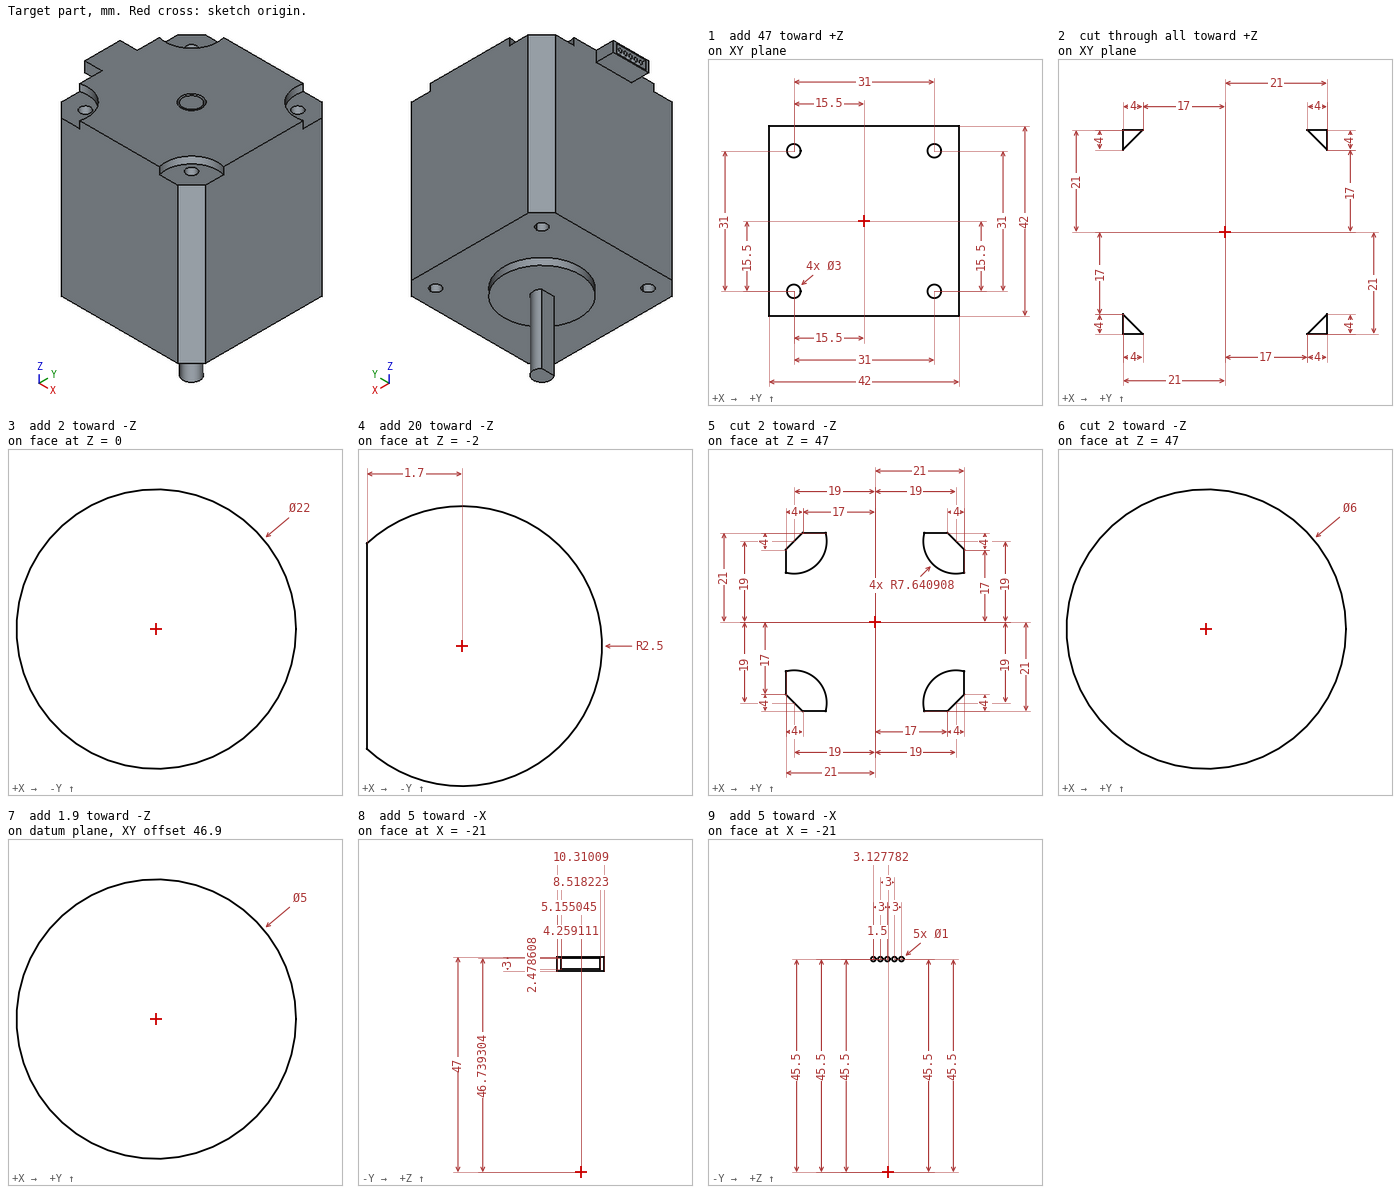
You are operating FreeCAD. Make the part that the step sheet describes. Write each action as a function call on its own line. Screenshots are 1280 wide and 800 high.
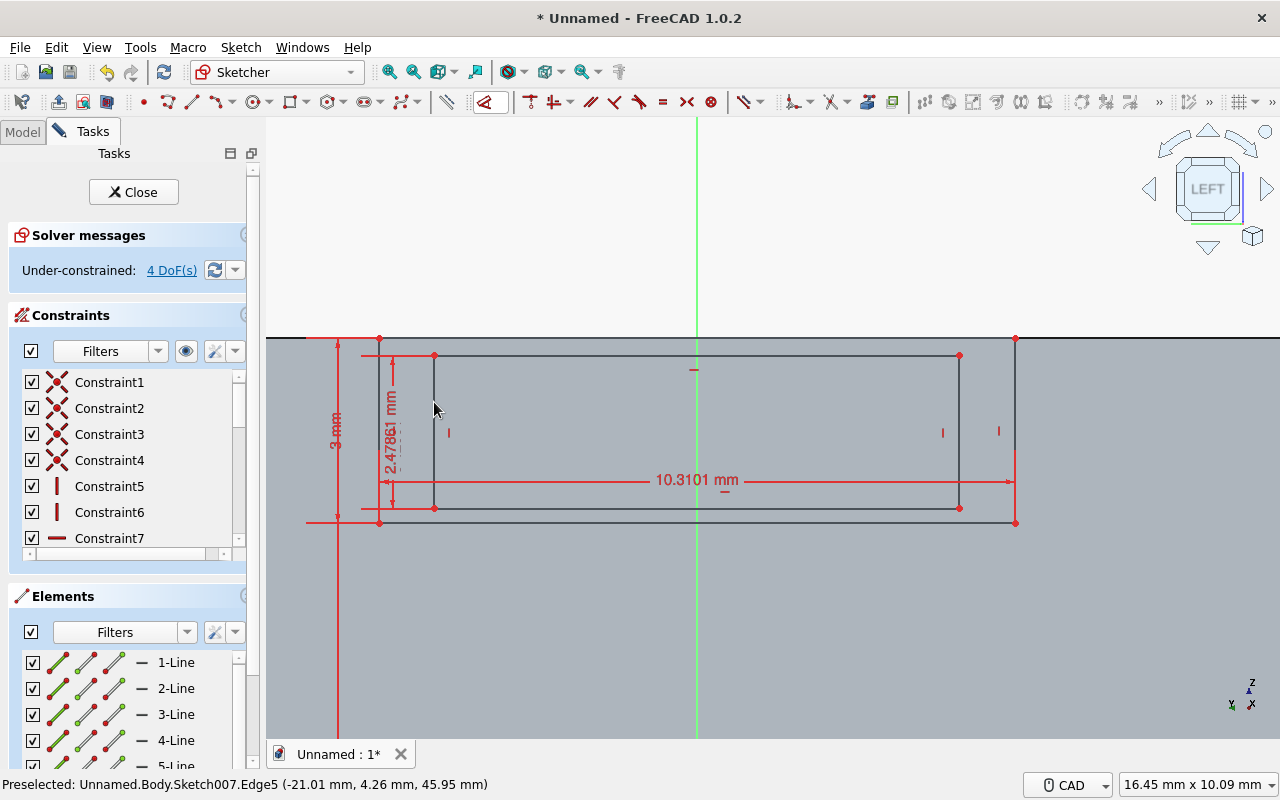
click(591, 509)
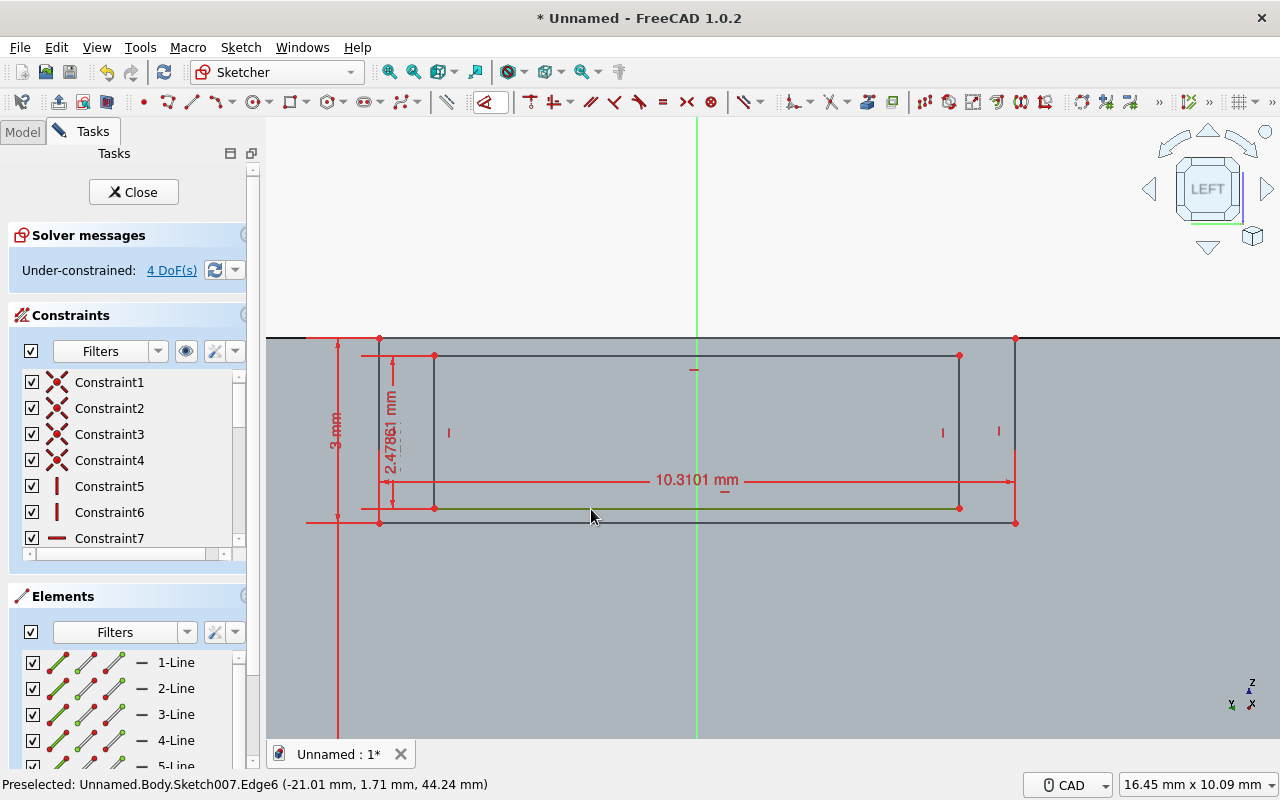
key(l)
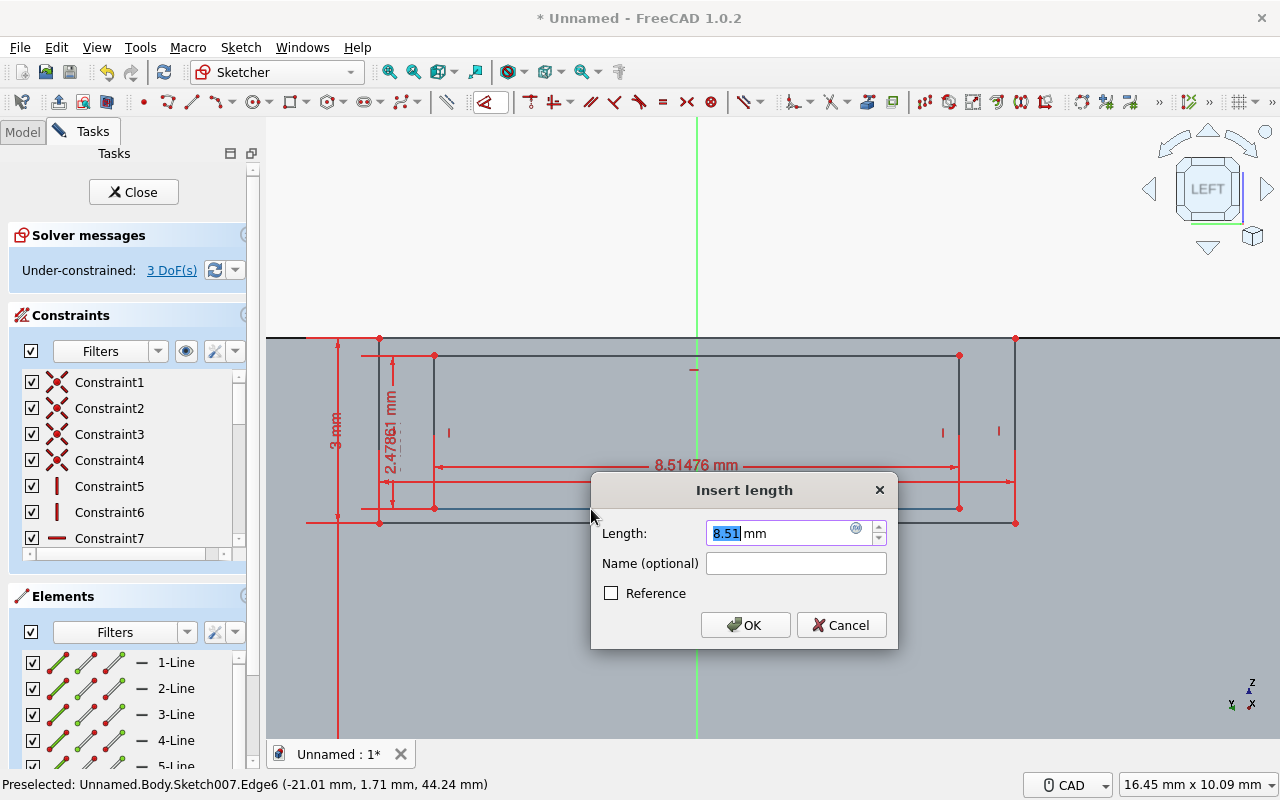
text(8.518223)
key(Return)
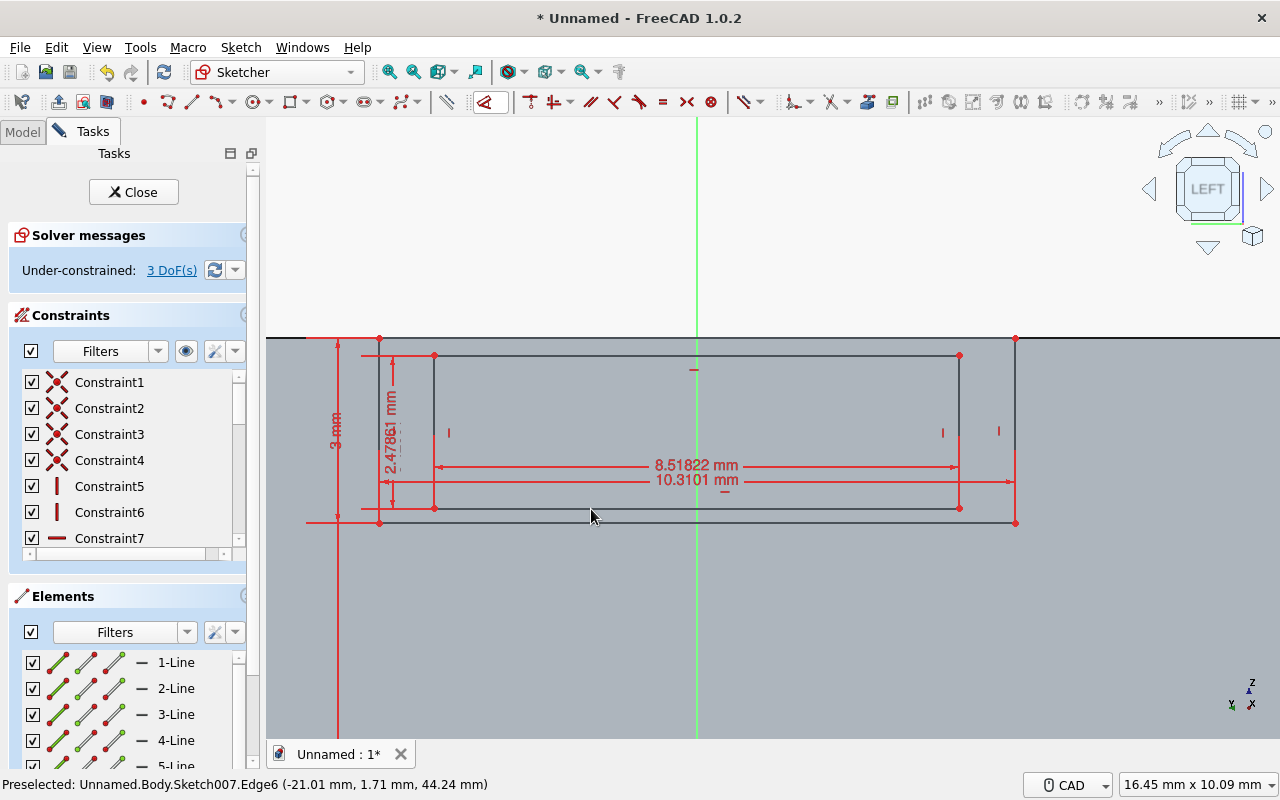
click(379, 338)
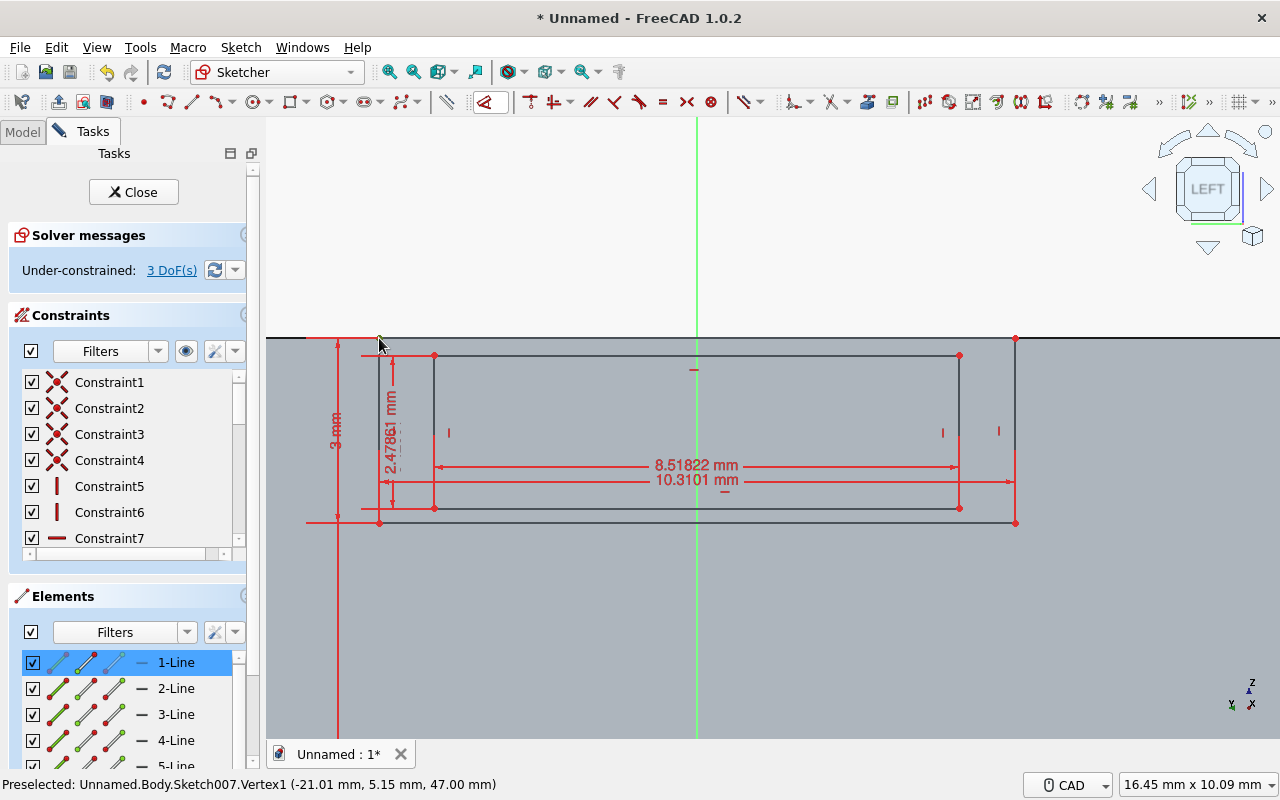
click(502, 102)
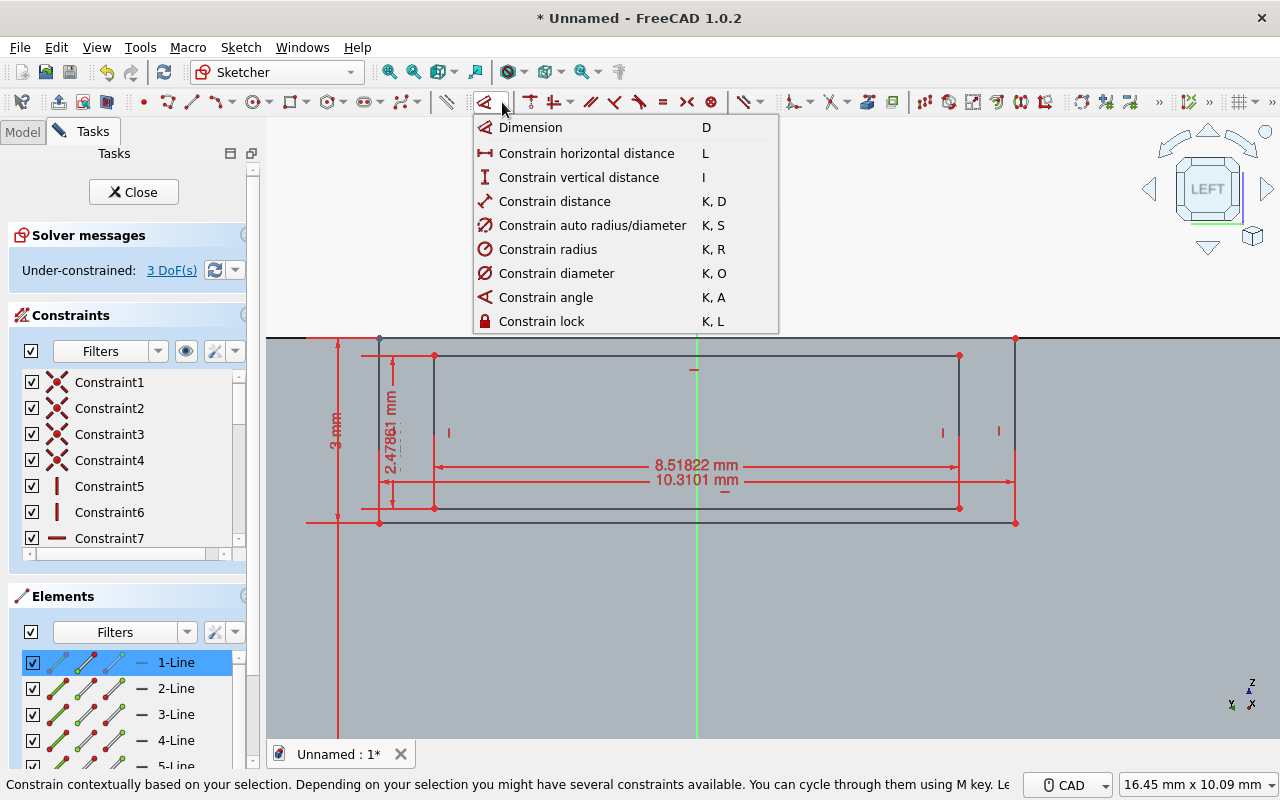
click(626, 153)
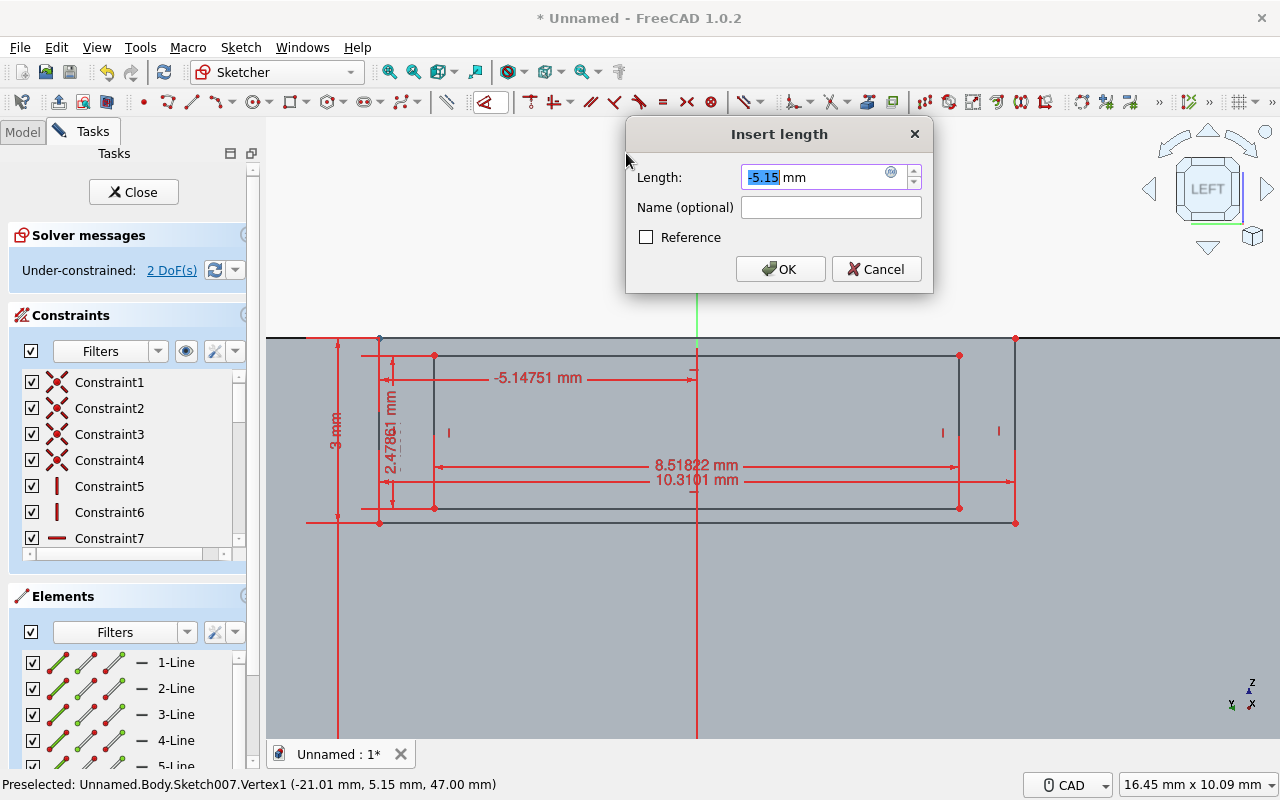
text(-5.155045)
key(Return)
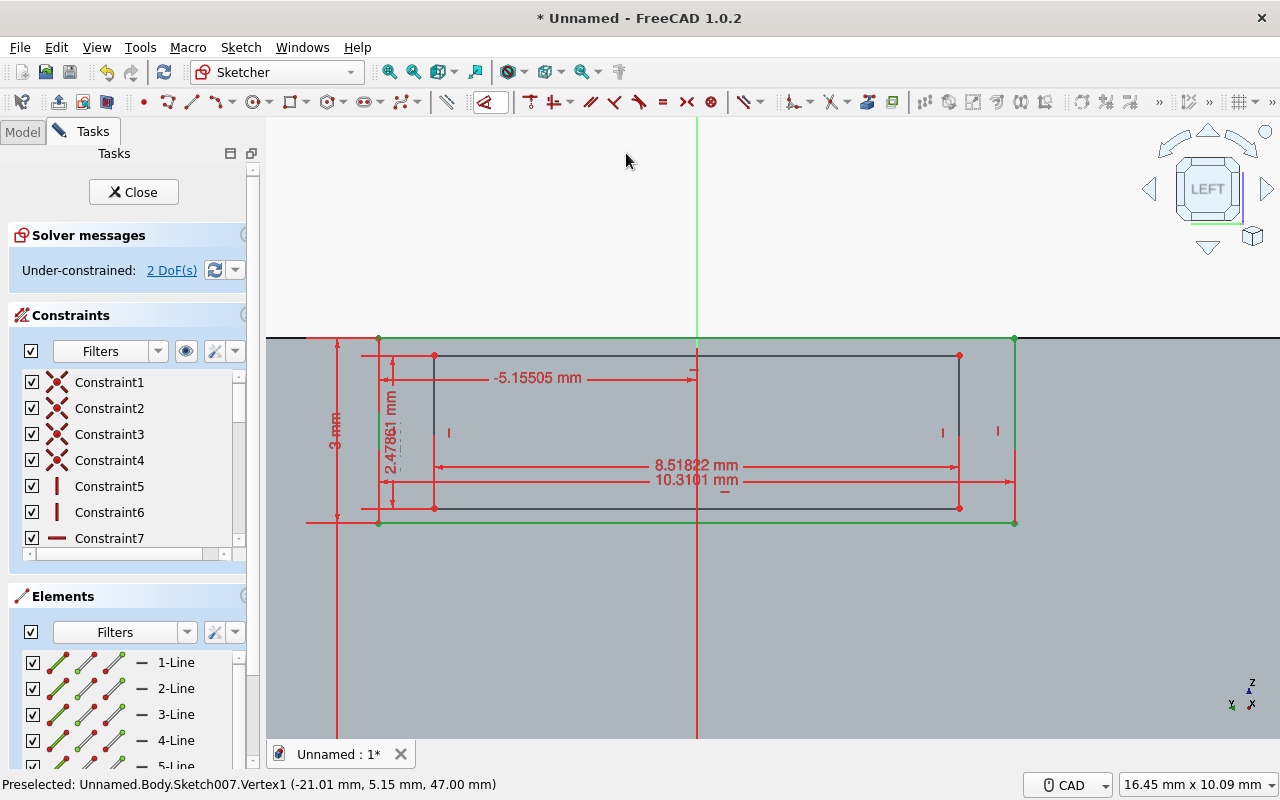
click(434, 356)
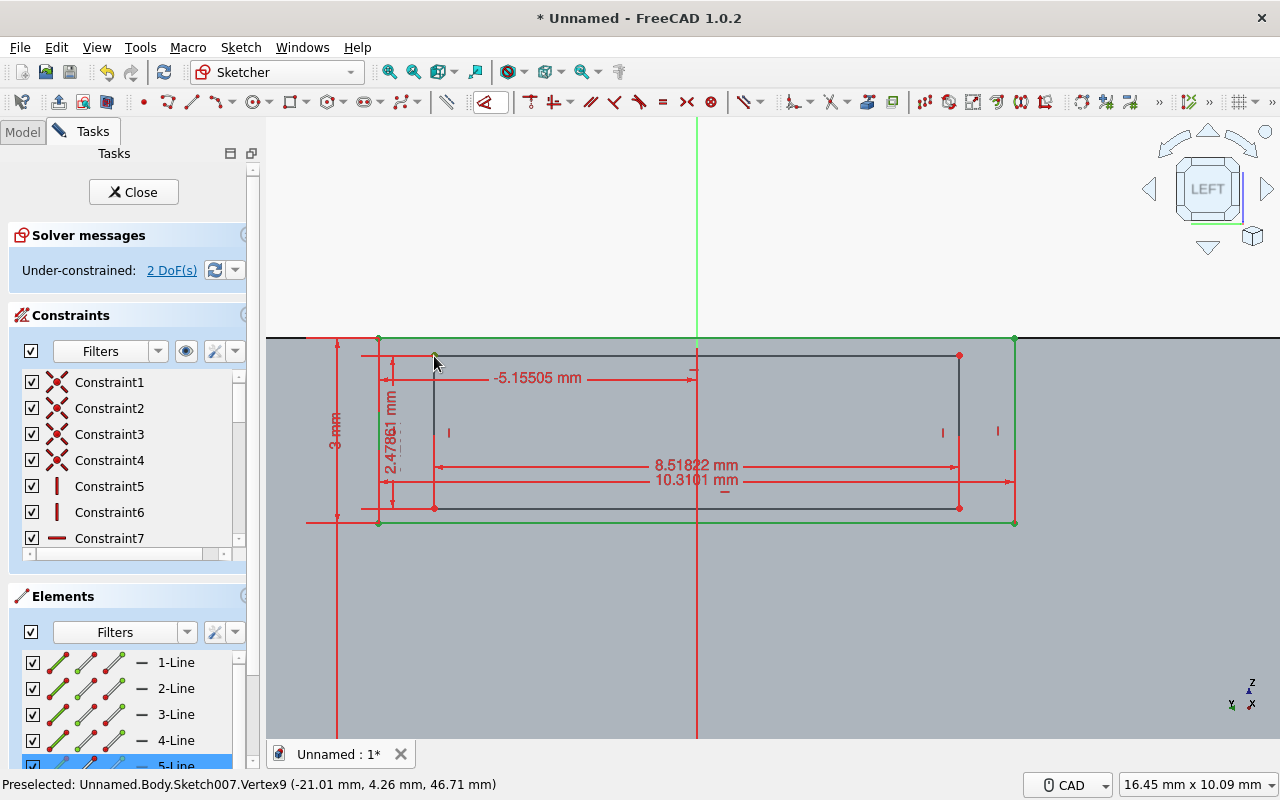
key(l)